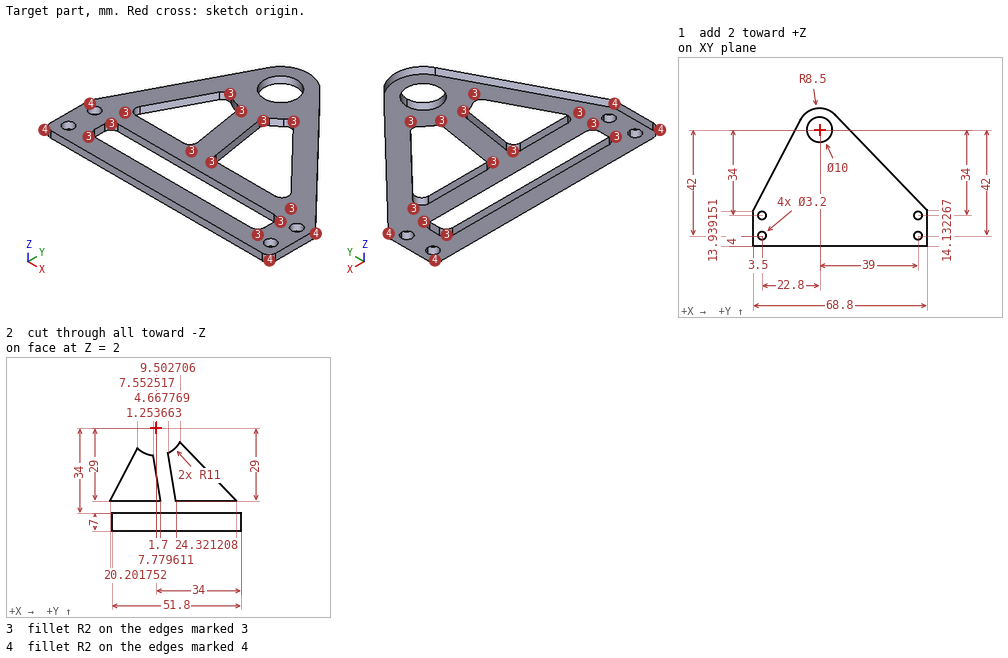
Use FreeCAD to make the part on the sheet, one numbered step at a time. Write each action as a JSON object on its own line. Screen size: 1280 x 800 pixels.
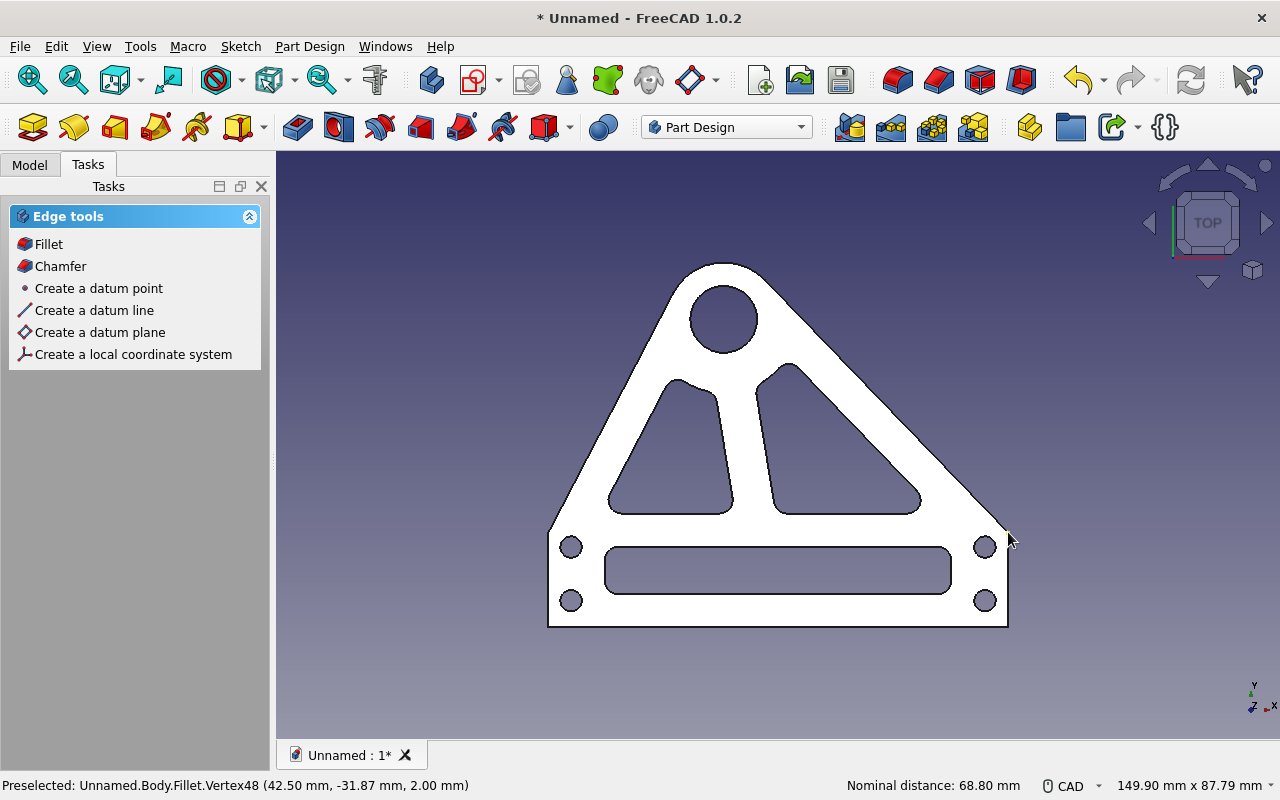
{"action": "key", "text": "1"}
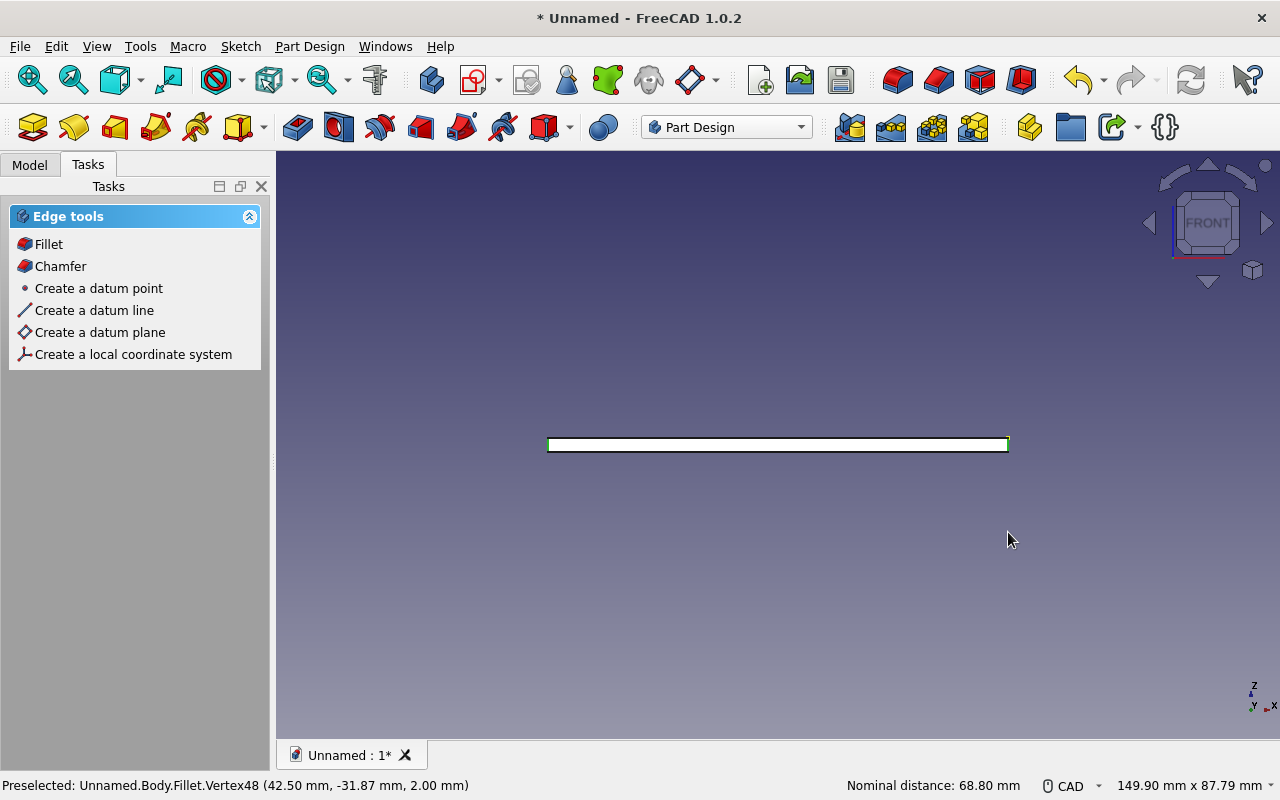
{"action": "scroll", "coordinate": [1008, 444], "scroll_direction": "up", "scroll_amount": 6}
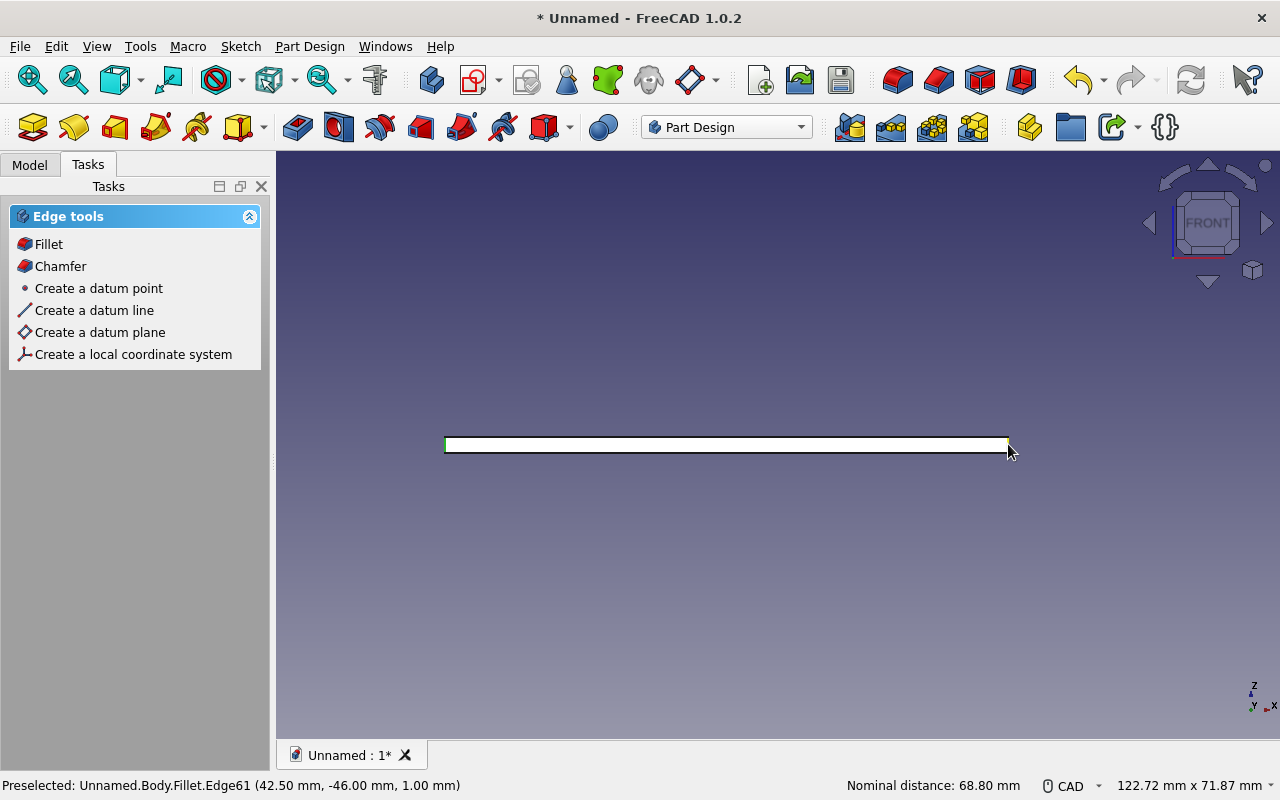
{"action": "left_click", "coordinate": [33, 80]}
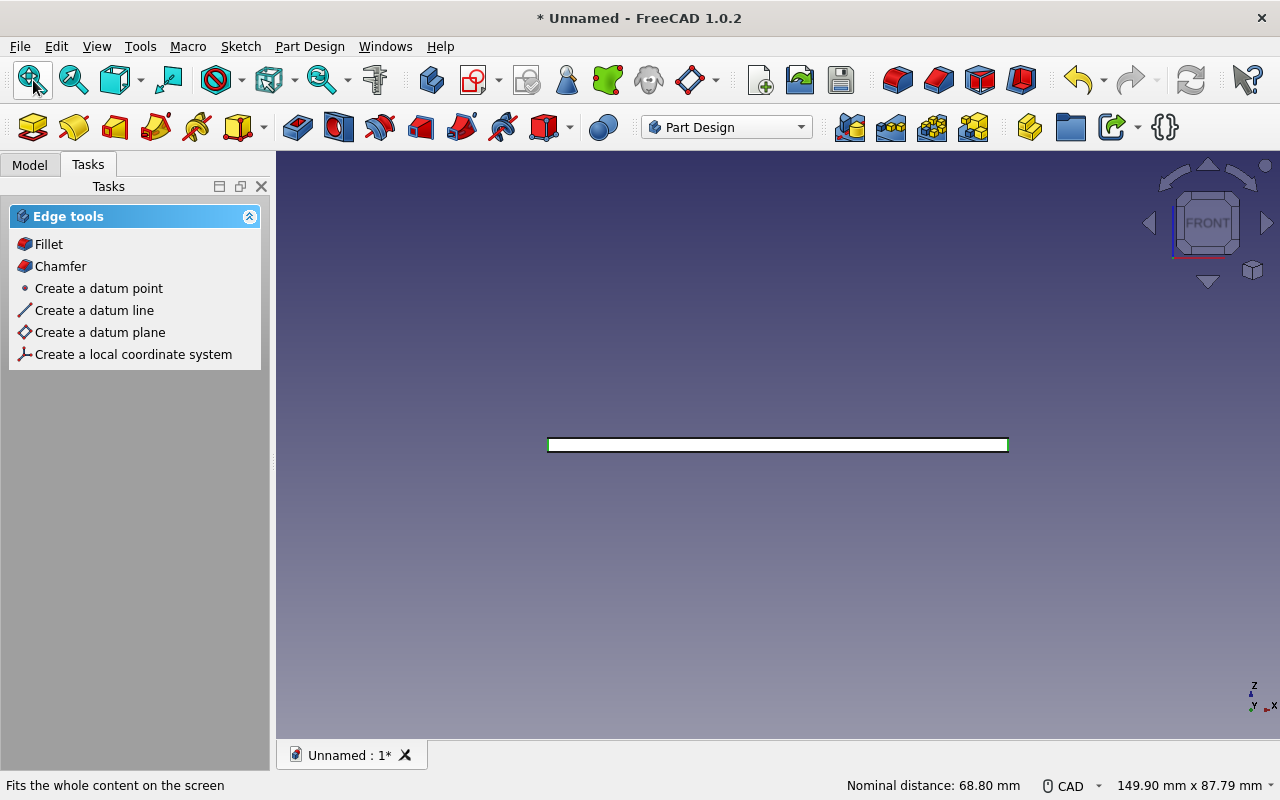
{"action": "key", "text": "3"}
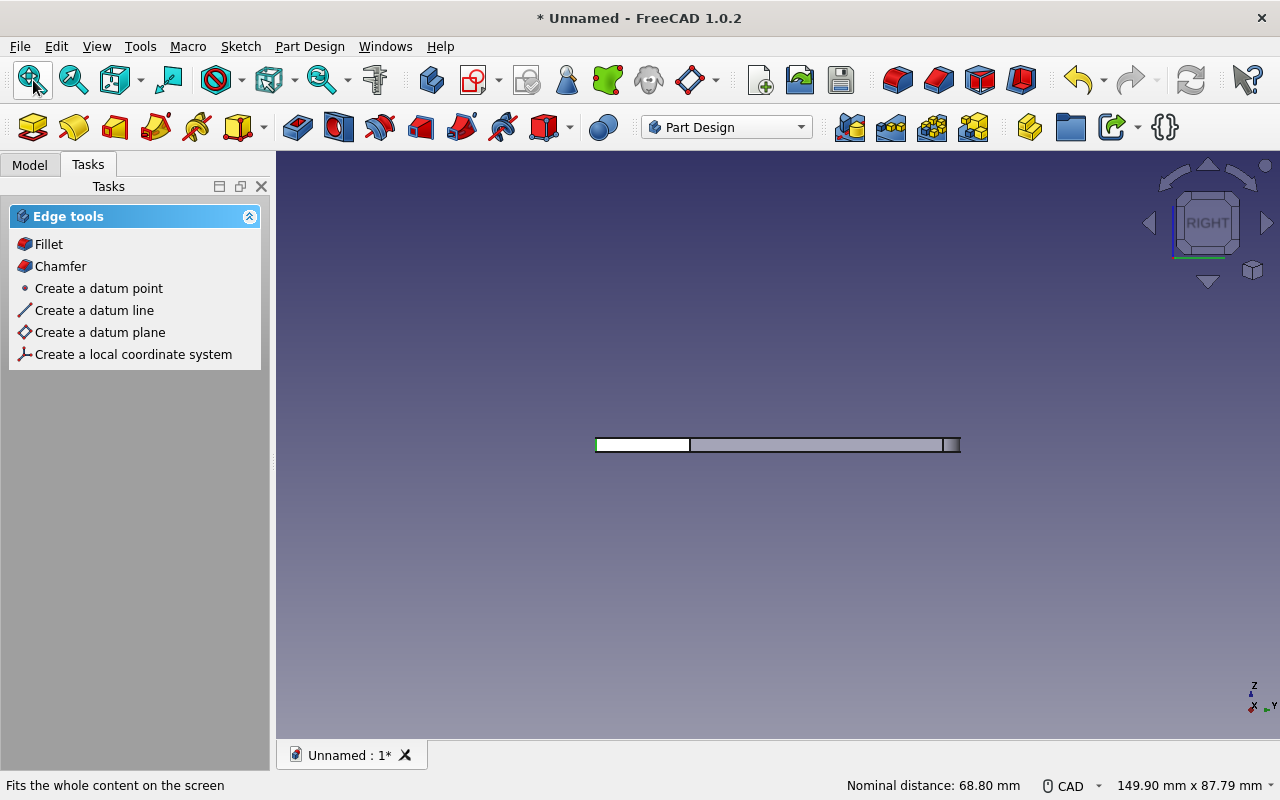
{"action": "left_click", "coordinate": [33, 80]}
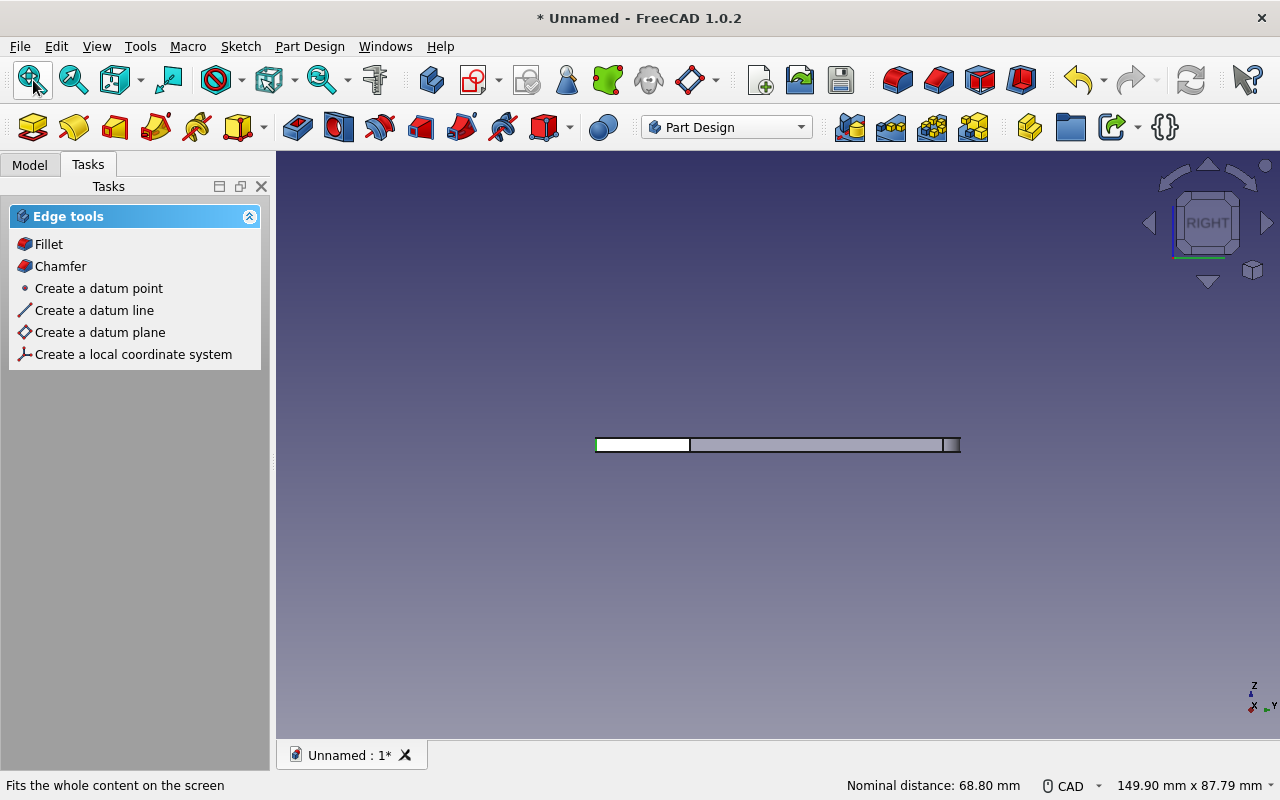
{"action": "left_click", "coordinate": [690, 444], "text": "ctrl"}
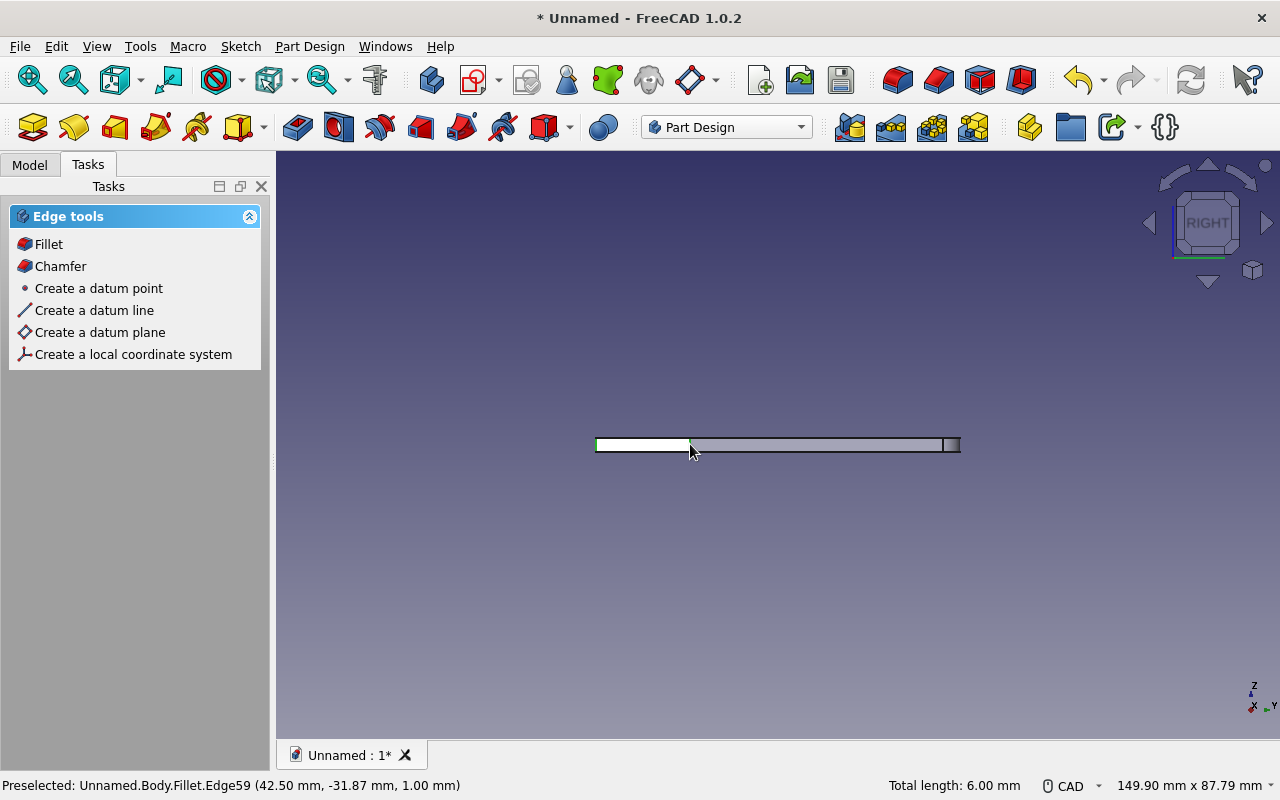
{"action": "scroll", "coordinate": [689, 444], "scroll_direction": "up", "scroll_amount": 6}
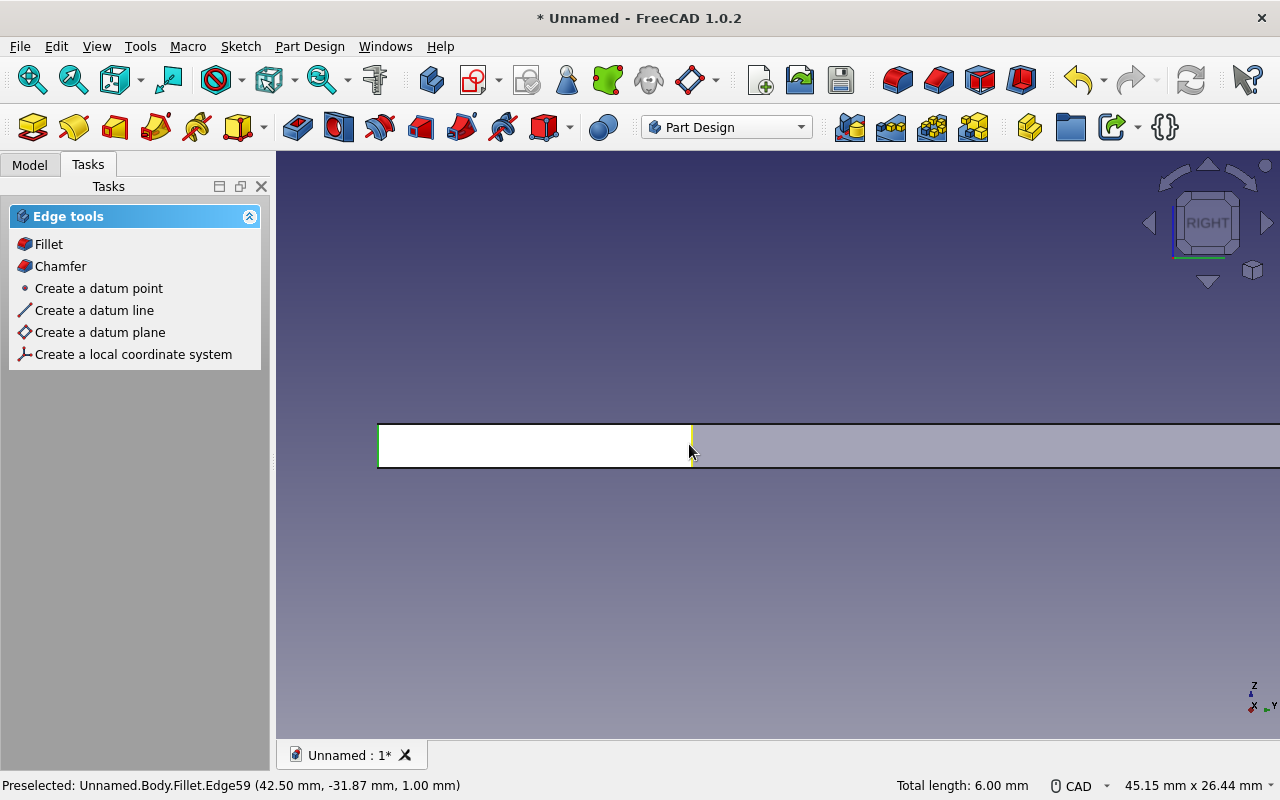
{"action": "left_click", "coordinate": [33, 80]}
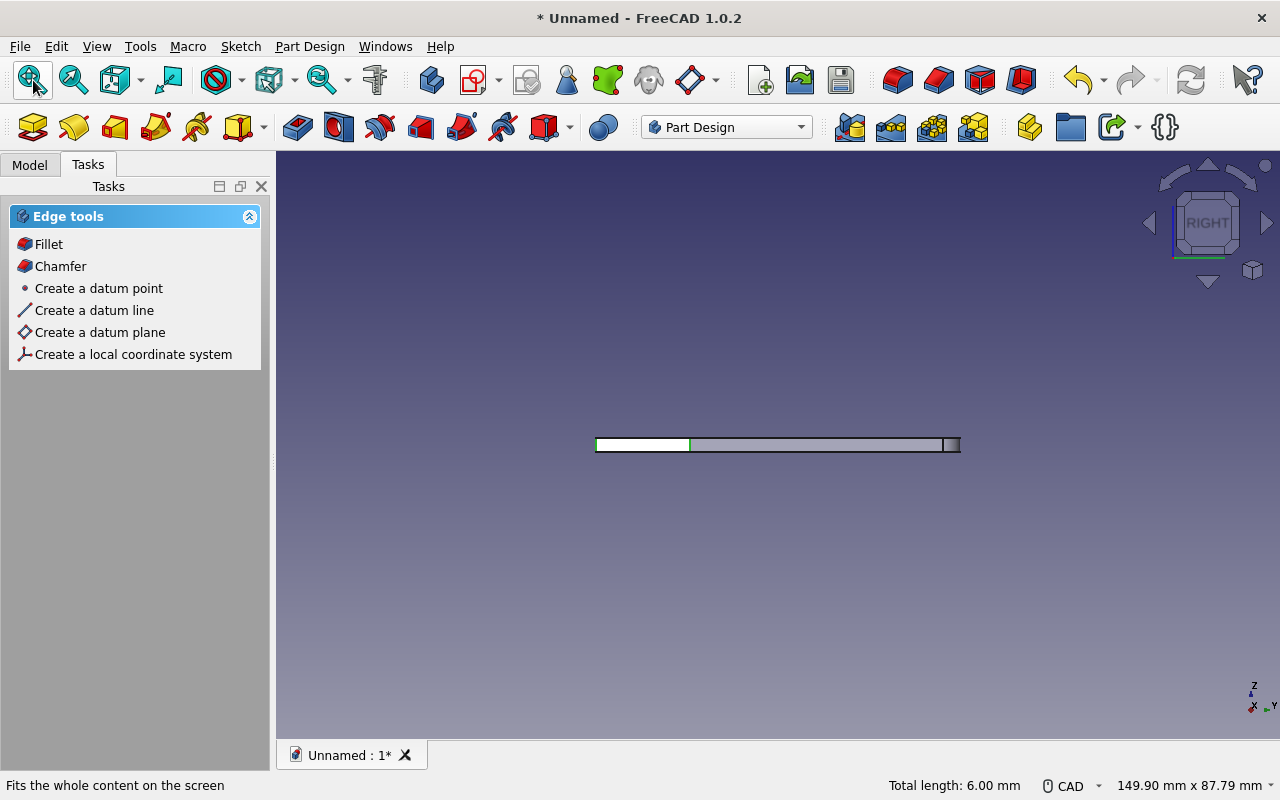
{"action": "key", "text": "5"}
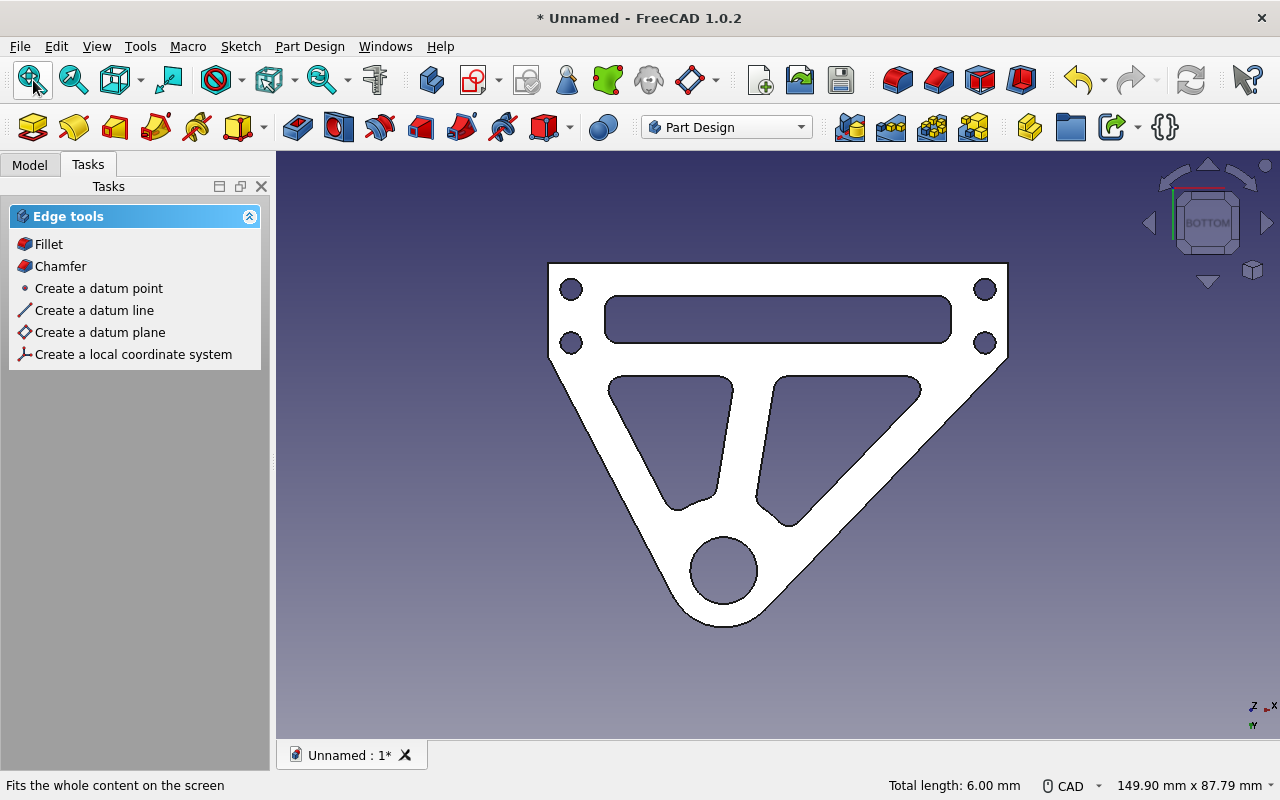
{"action": "scroll", "coordinate": [548, 355], "scroll_direction": "up", "scroll_amount": 6}